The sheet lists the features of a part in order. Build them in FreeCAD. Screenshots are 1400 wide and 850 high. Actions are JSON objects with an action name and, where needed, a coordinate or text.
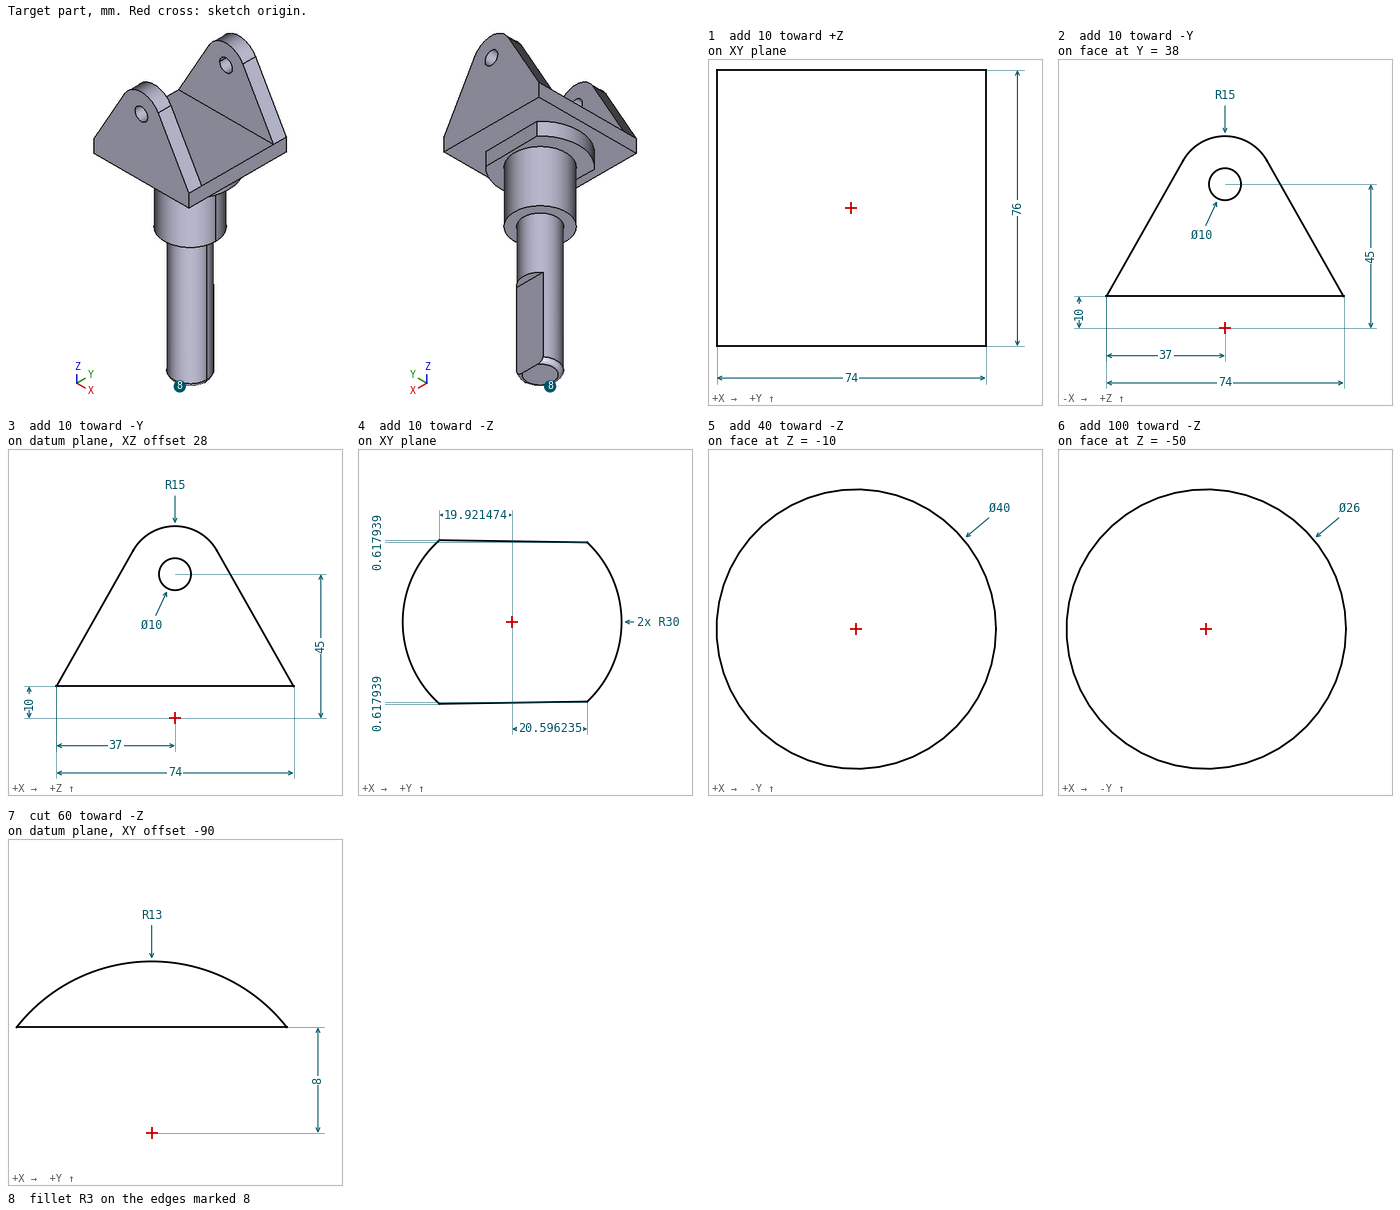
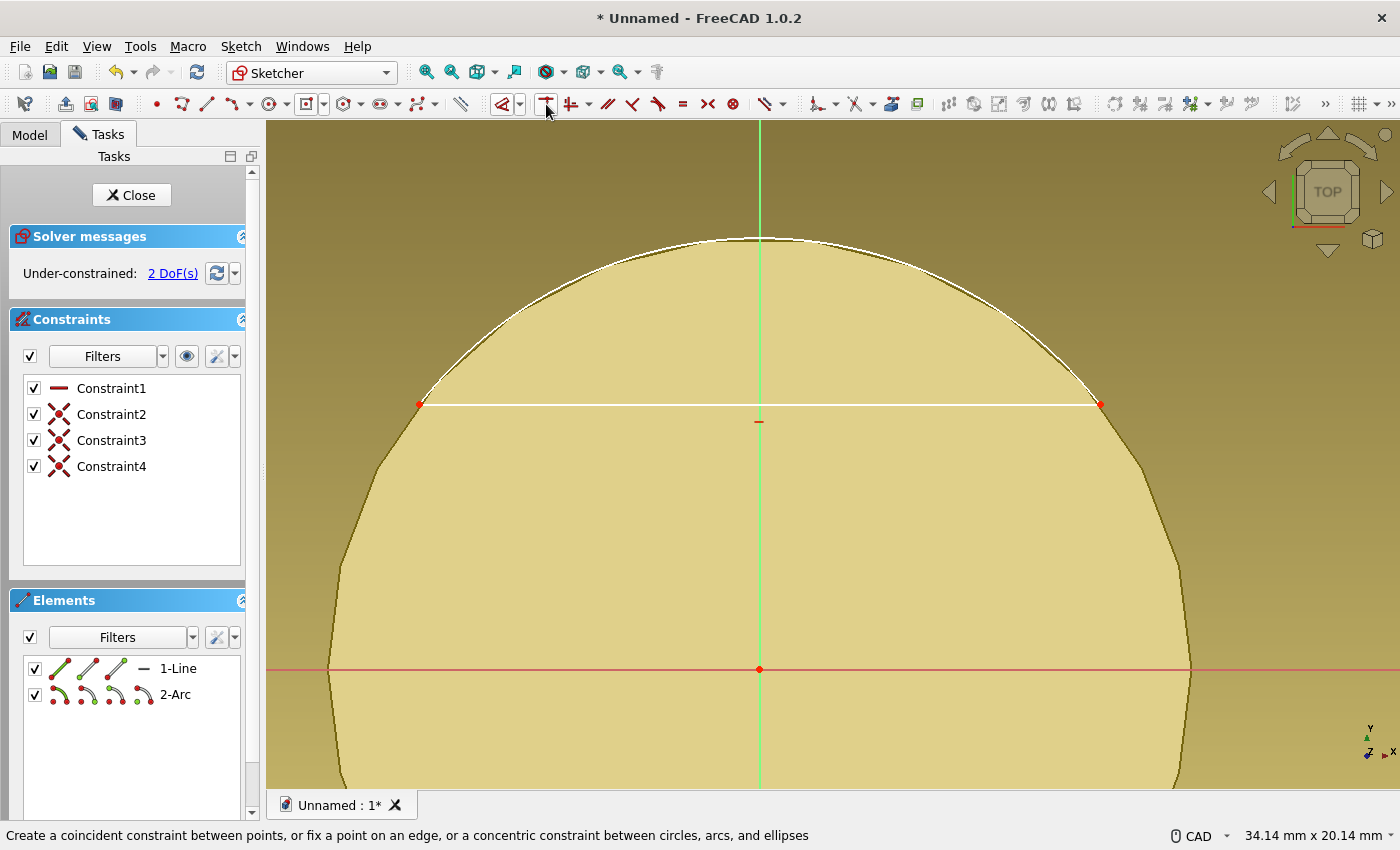
{"action": "left_click", "coordinate": [913, 267]}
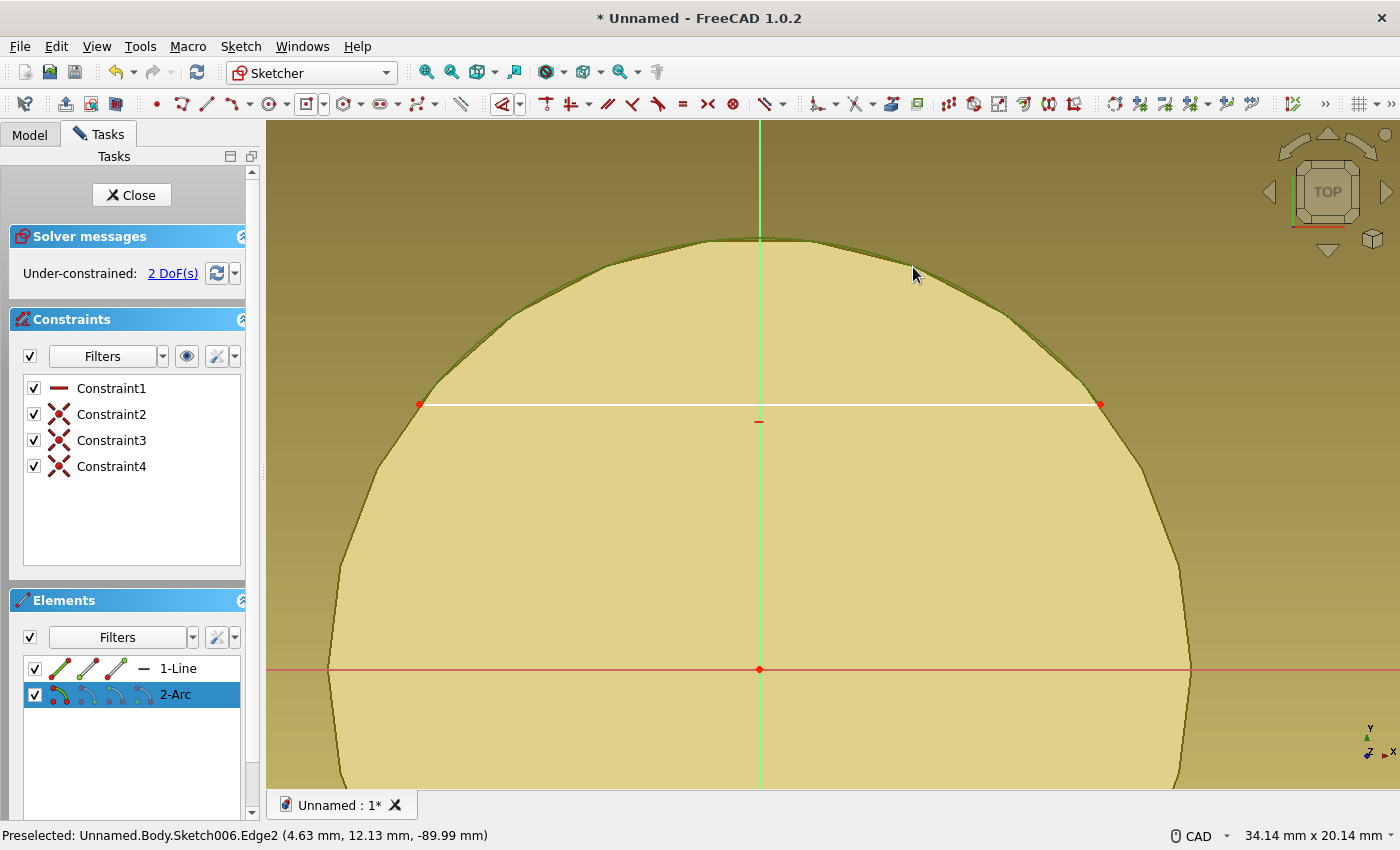
{"action": "left_click", "coordinate": [520, 104]}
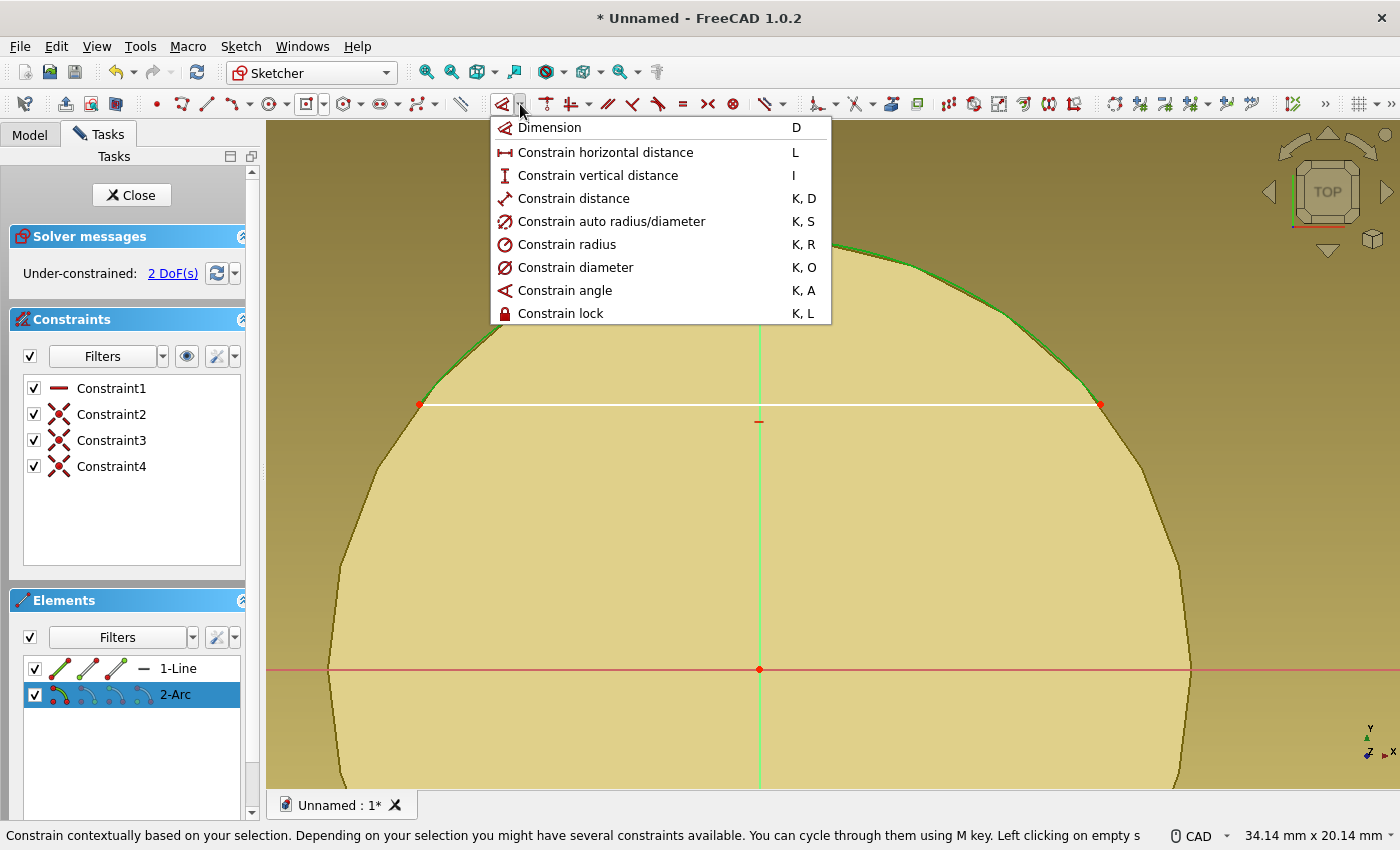
{"action": "left_click", "coordinate": [661, 244]}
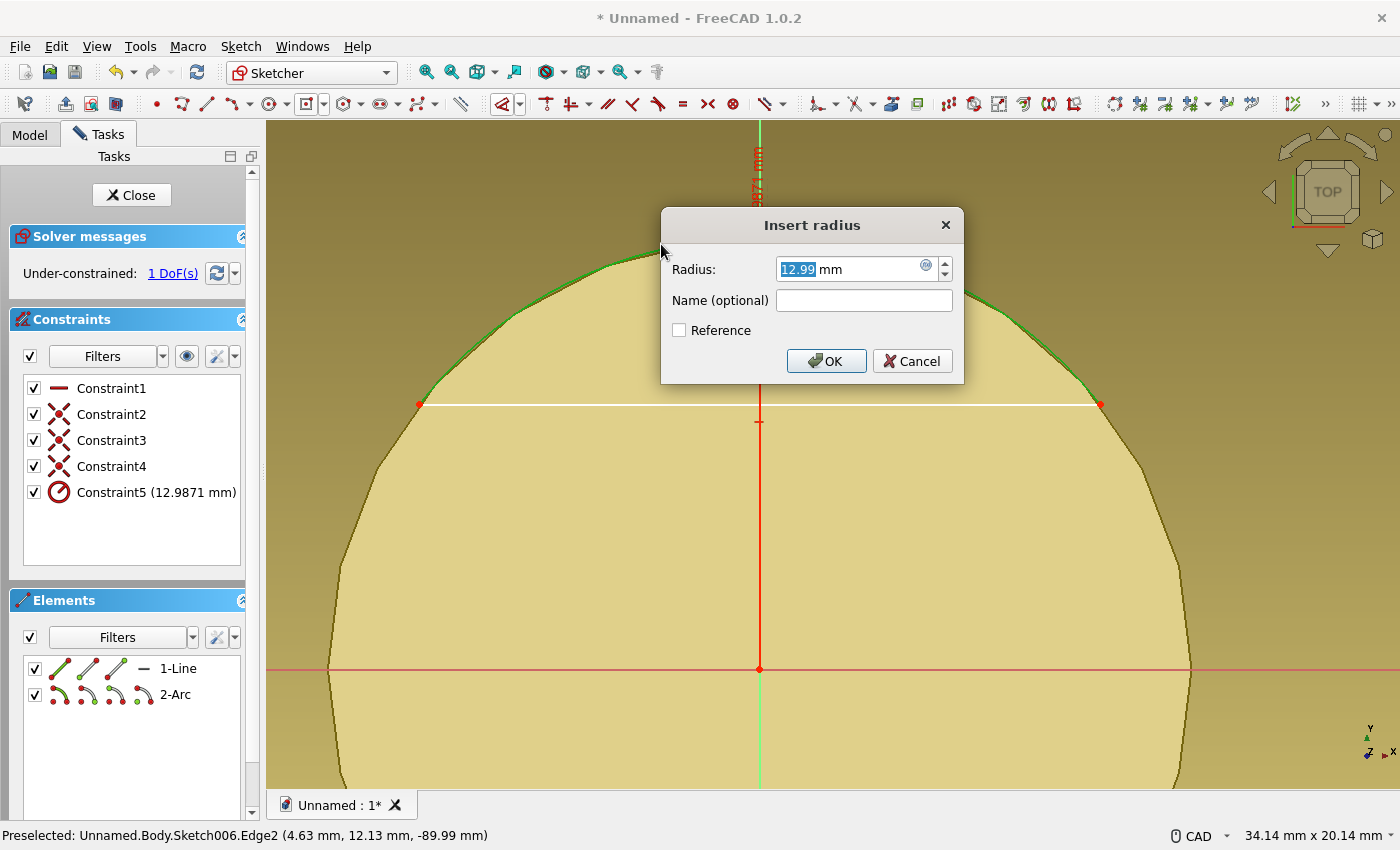
{"action": "type", "text": "13"}
{"action": "key", "text": "Return"}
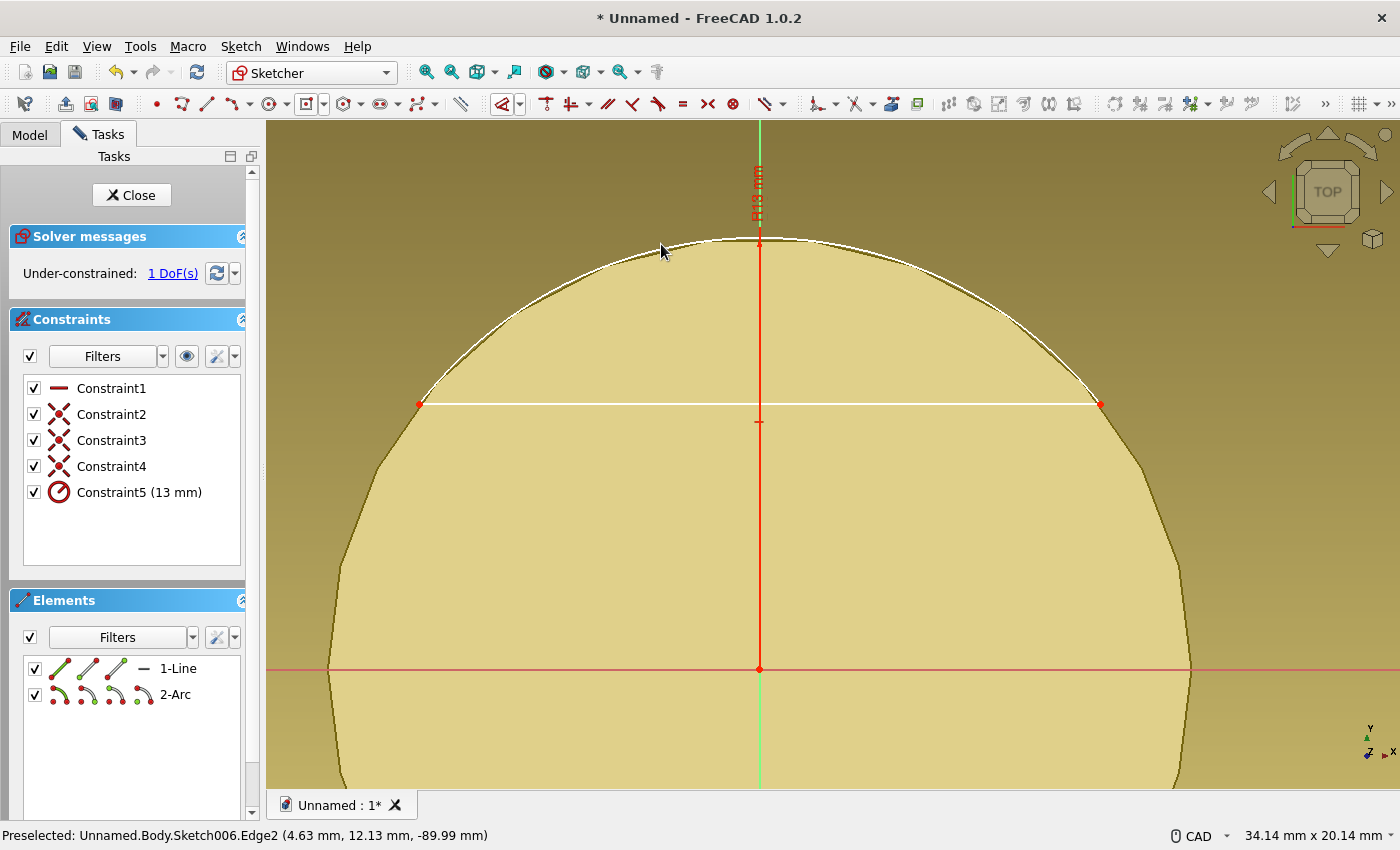
{"action": "left_click", "coordinate": [1100, 404]}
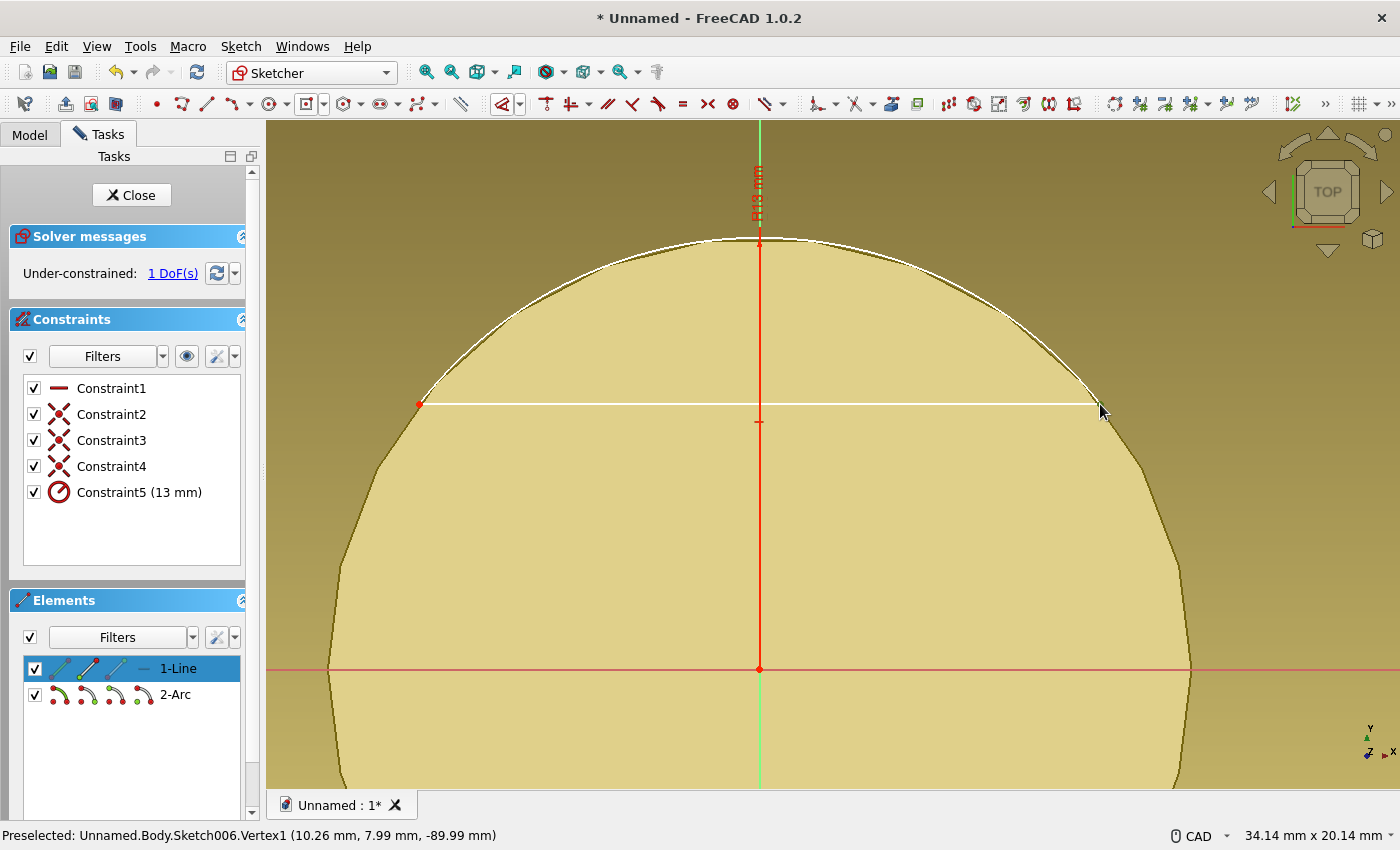
{"action": "key", "text": "i"}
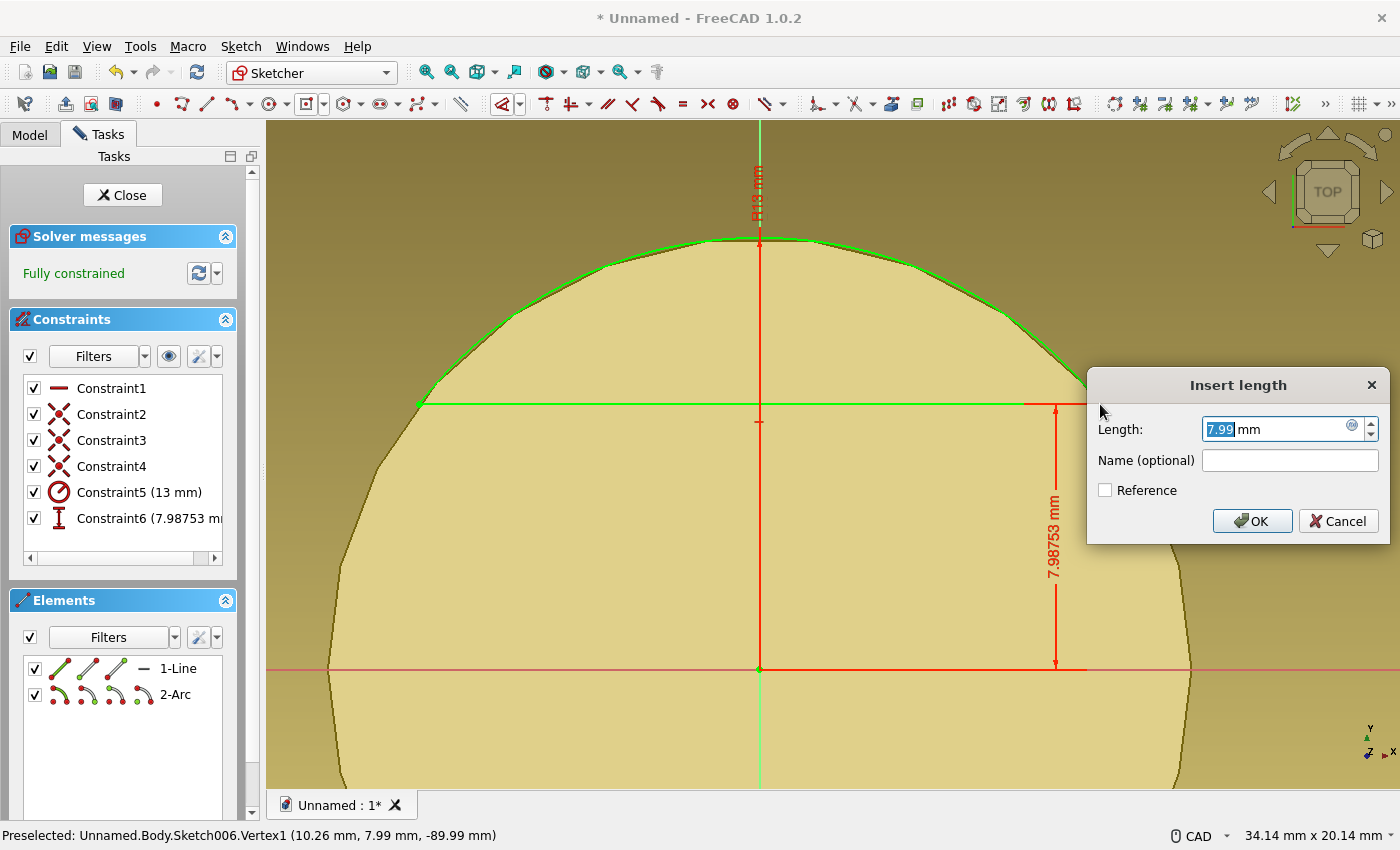
{"action": "type", "text": "8"}
{"action": "key", "text": "Return"}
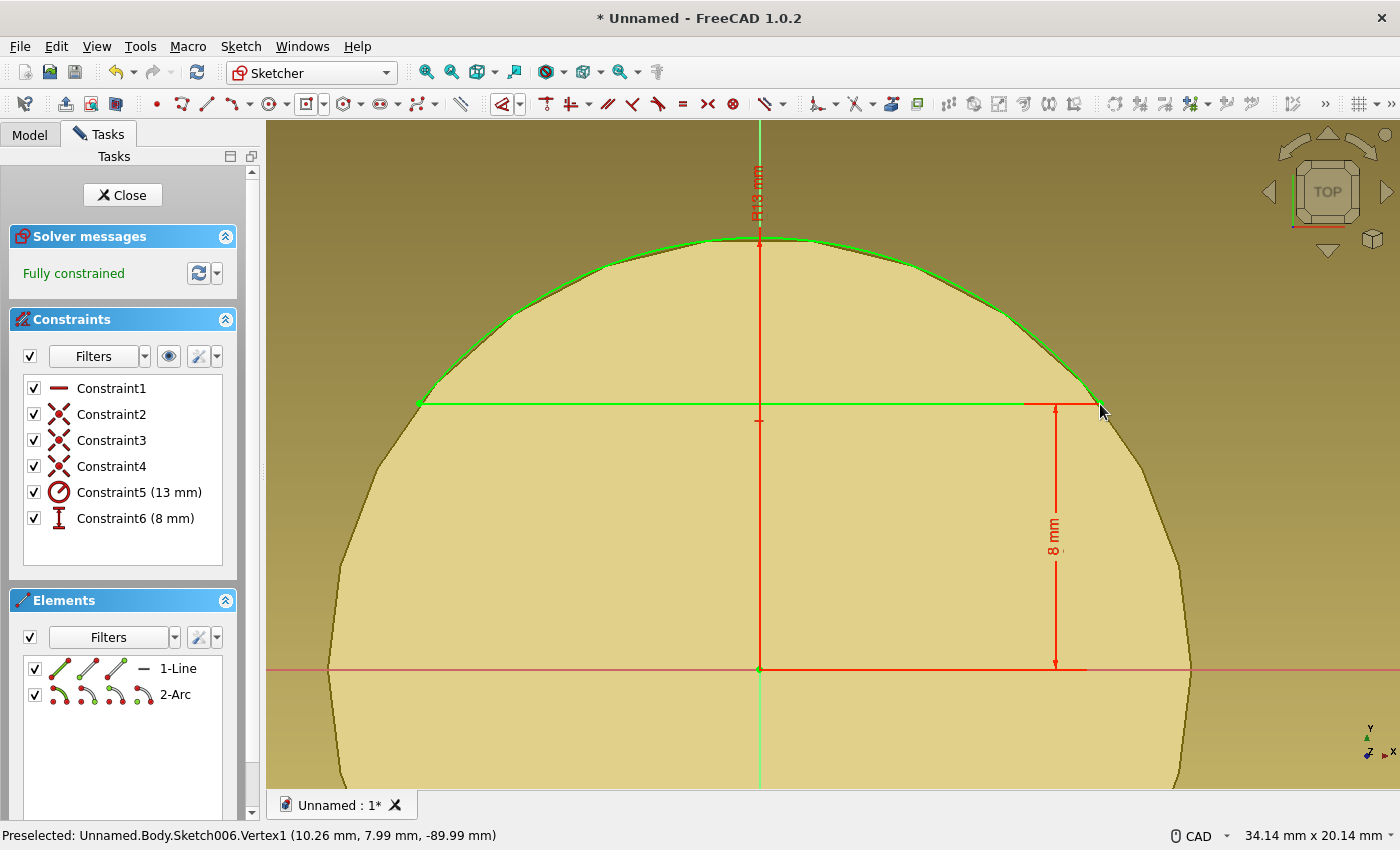
{"action": "left_click", "coordinate": [123, 195]}